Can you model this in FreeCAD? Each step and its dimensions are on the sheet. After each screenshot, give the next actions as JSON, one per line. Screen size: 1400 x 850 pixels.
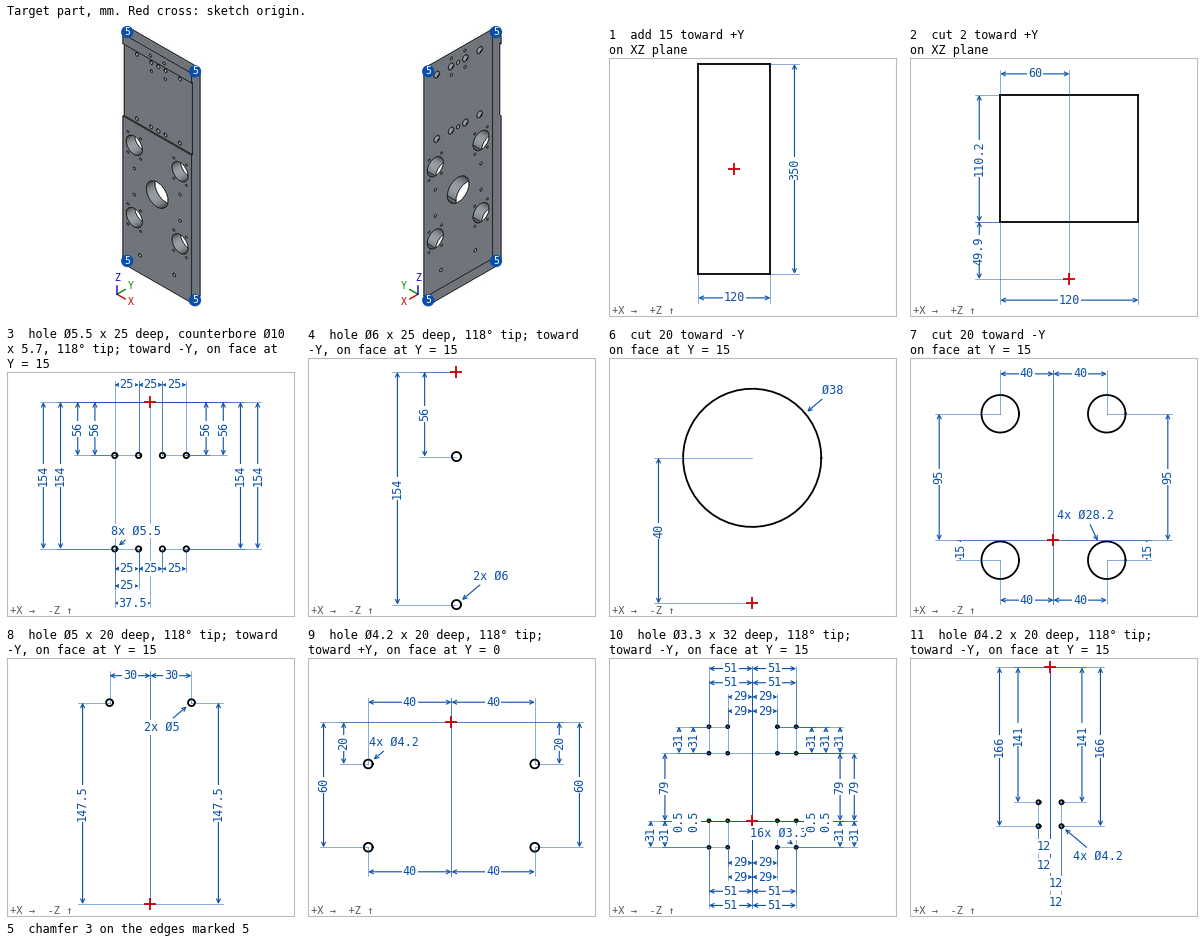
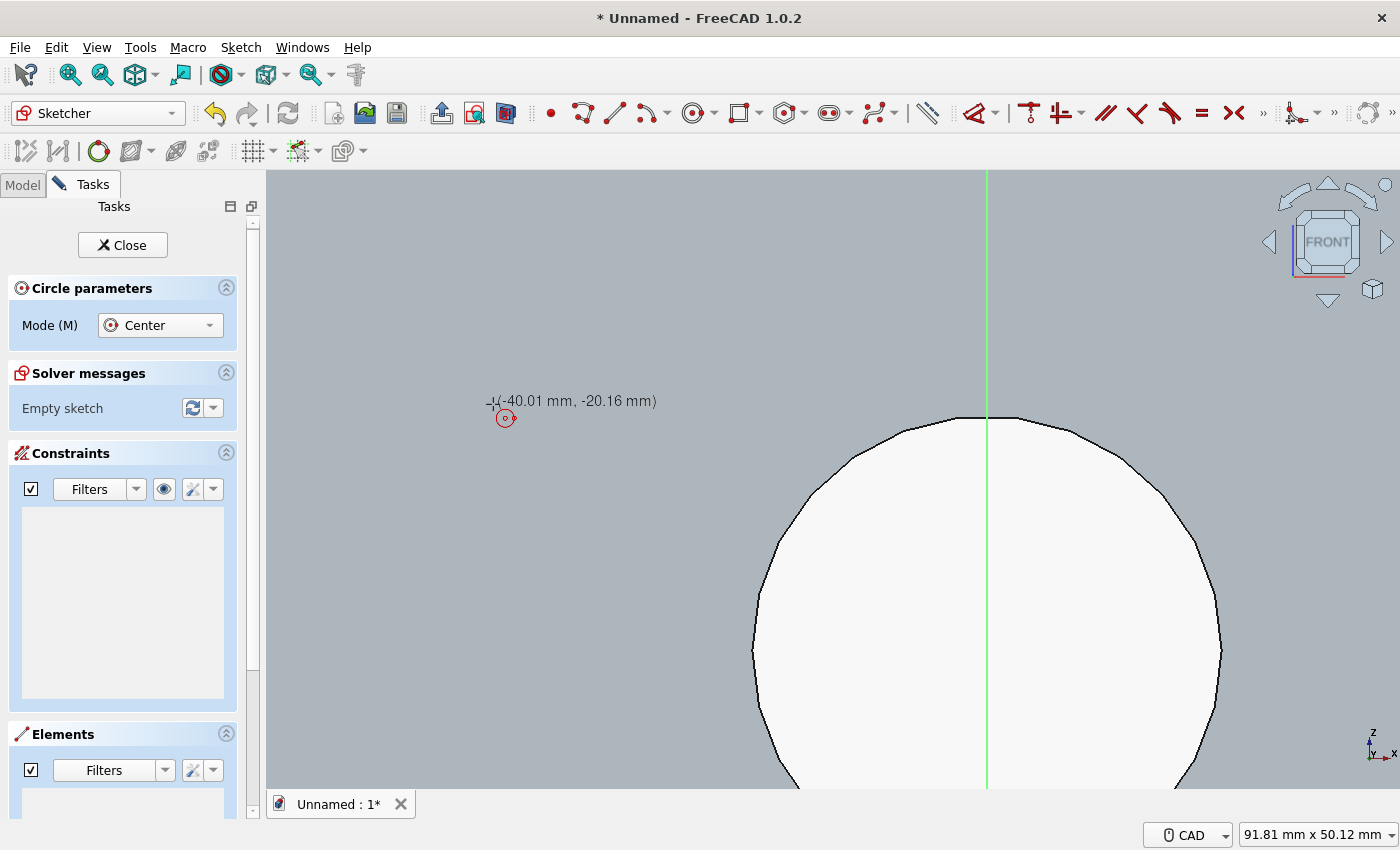
{"action": "left_click", "coordinate": [493, 404]}
{"action": "left_click", "coordinate": [511, 385]}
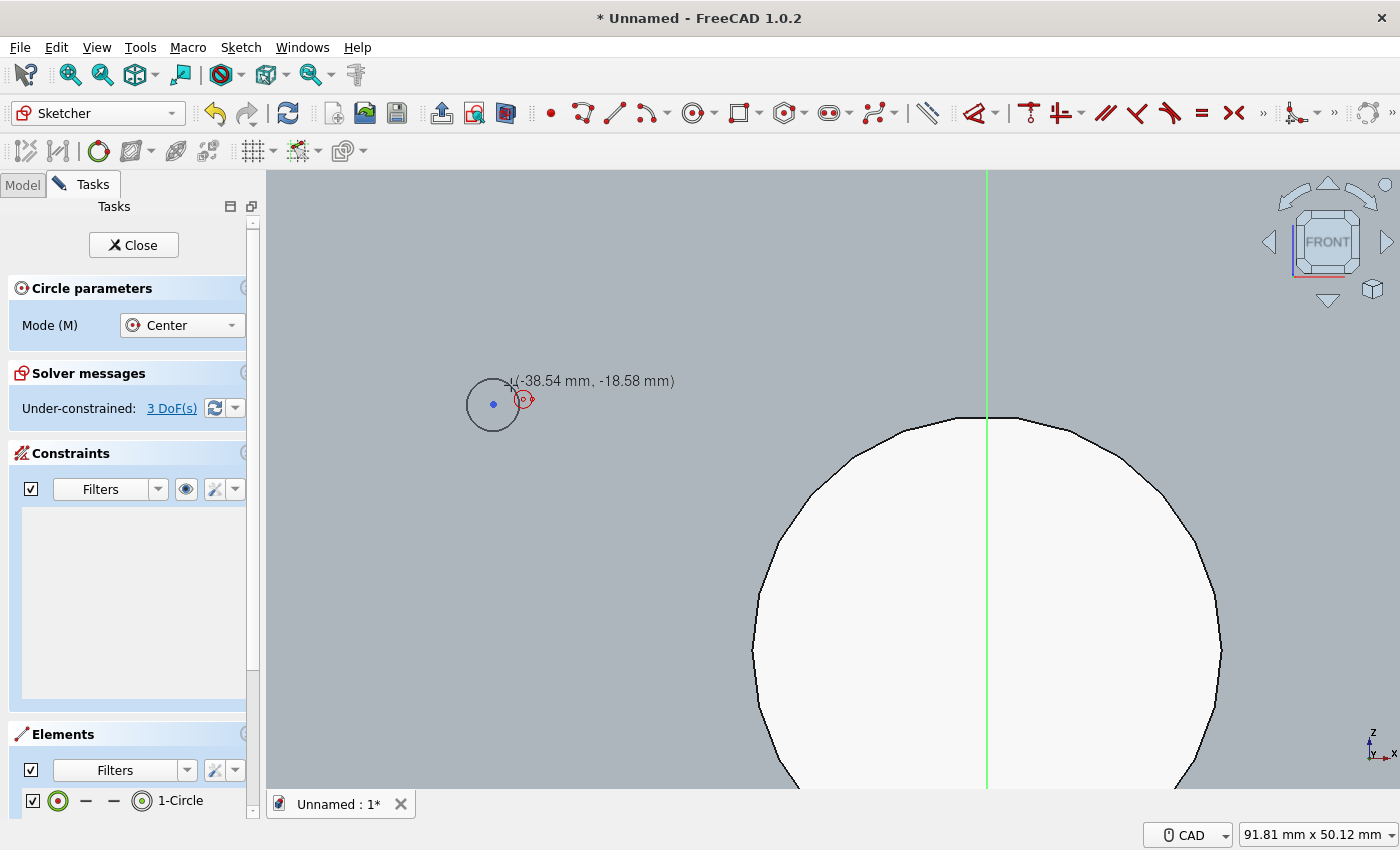
{"action": "scroll", "coordinate": [494, 406], "scroll_direction": "down", "scroll_amount": 3}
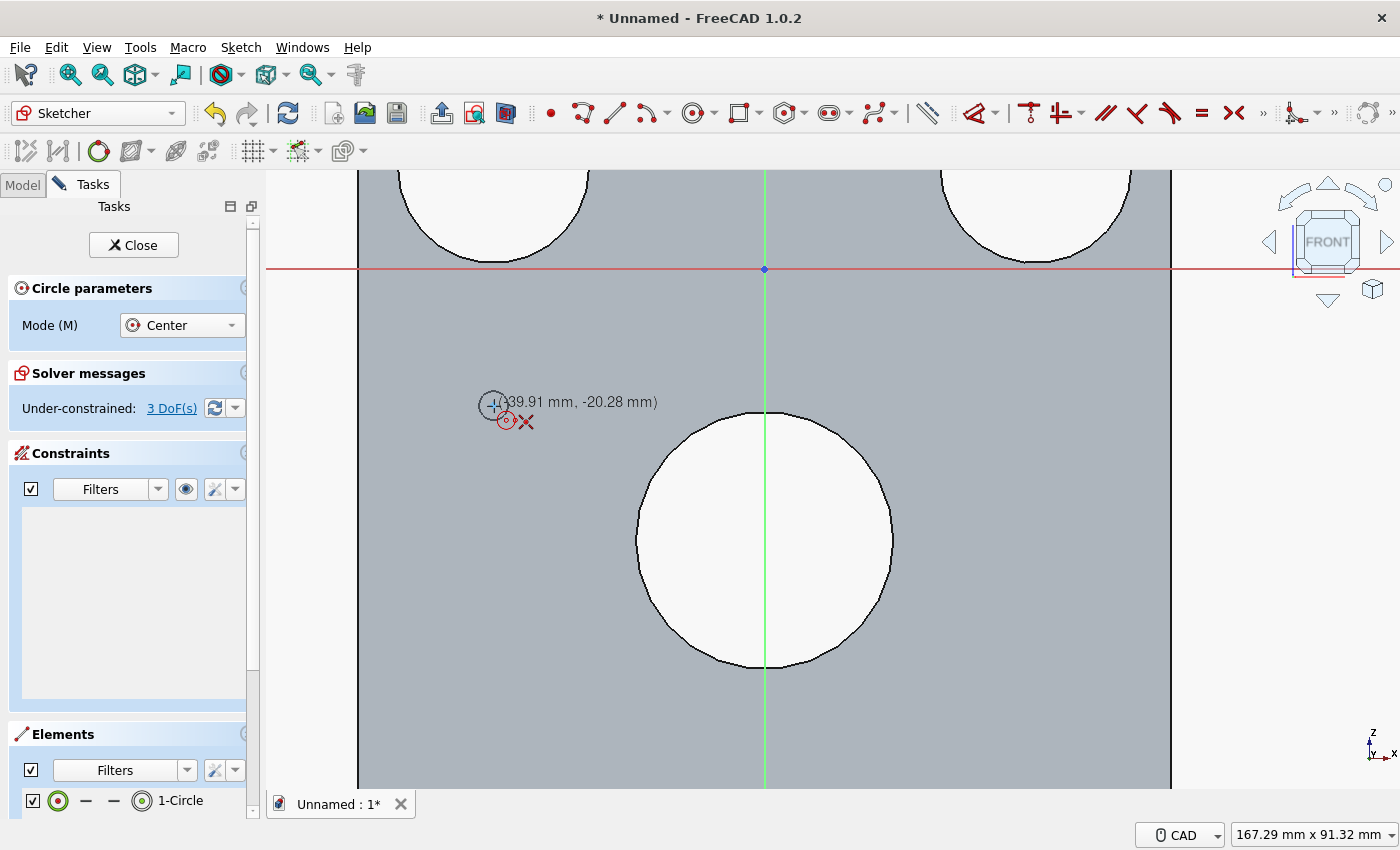
{"action": "scroll", "coordinate": [1036, 405], "scroll_direction": "up", "scroll_amount": 3}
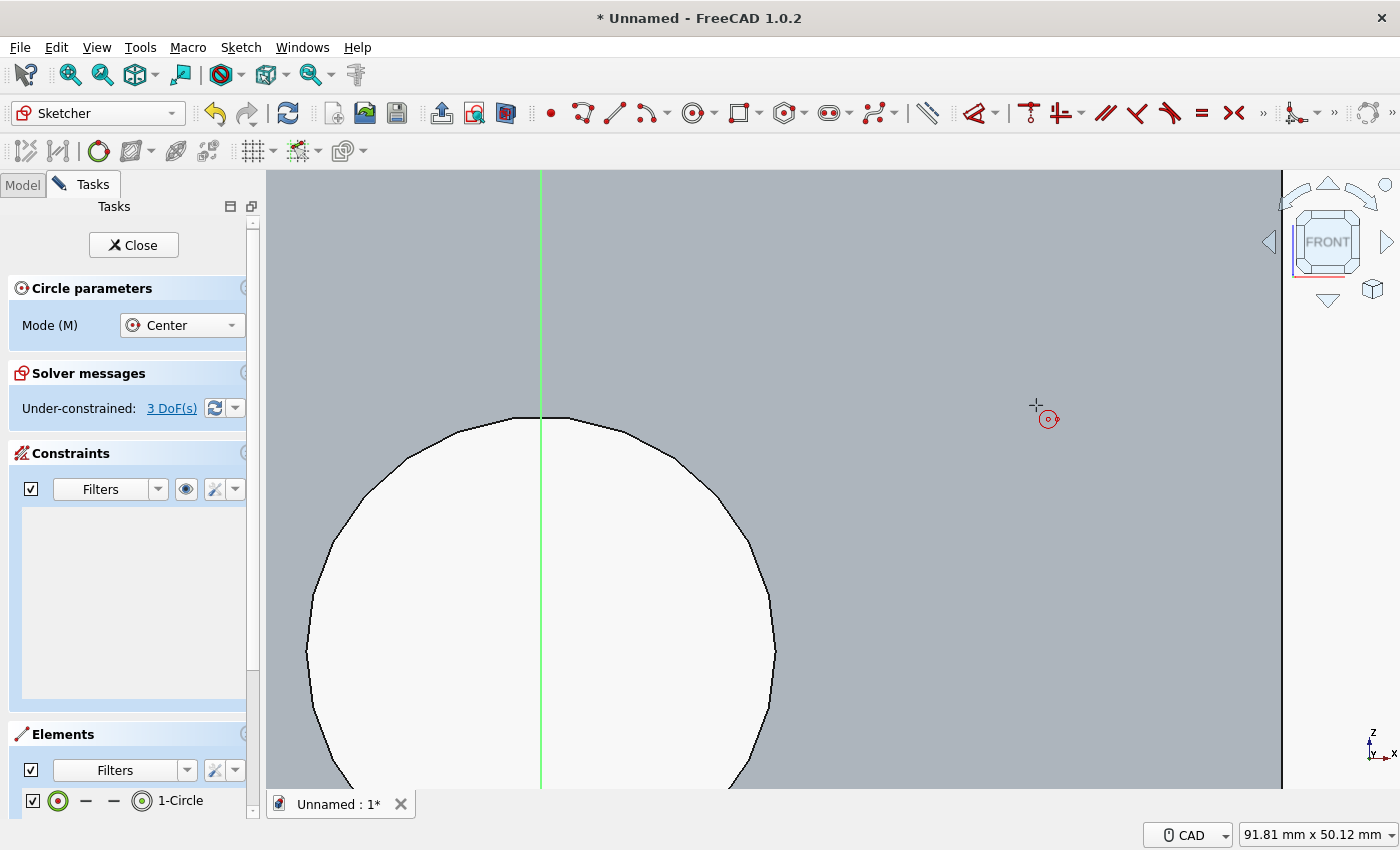
{"action": "left_click", "coordinate": [1035, 404]}
{"action": "left_click", "coordinate": [1053, 386]}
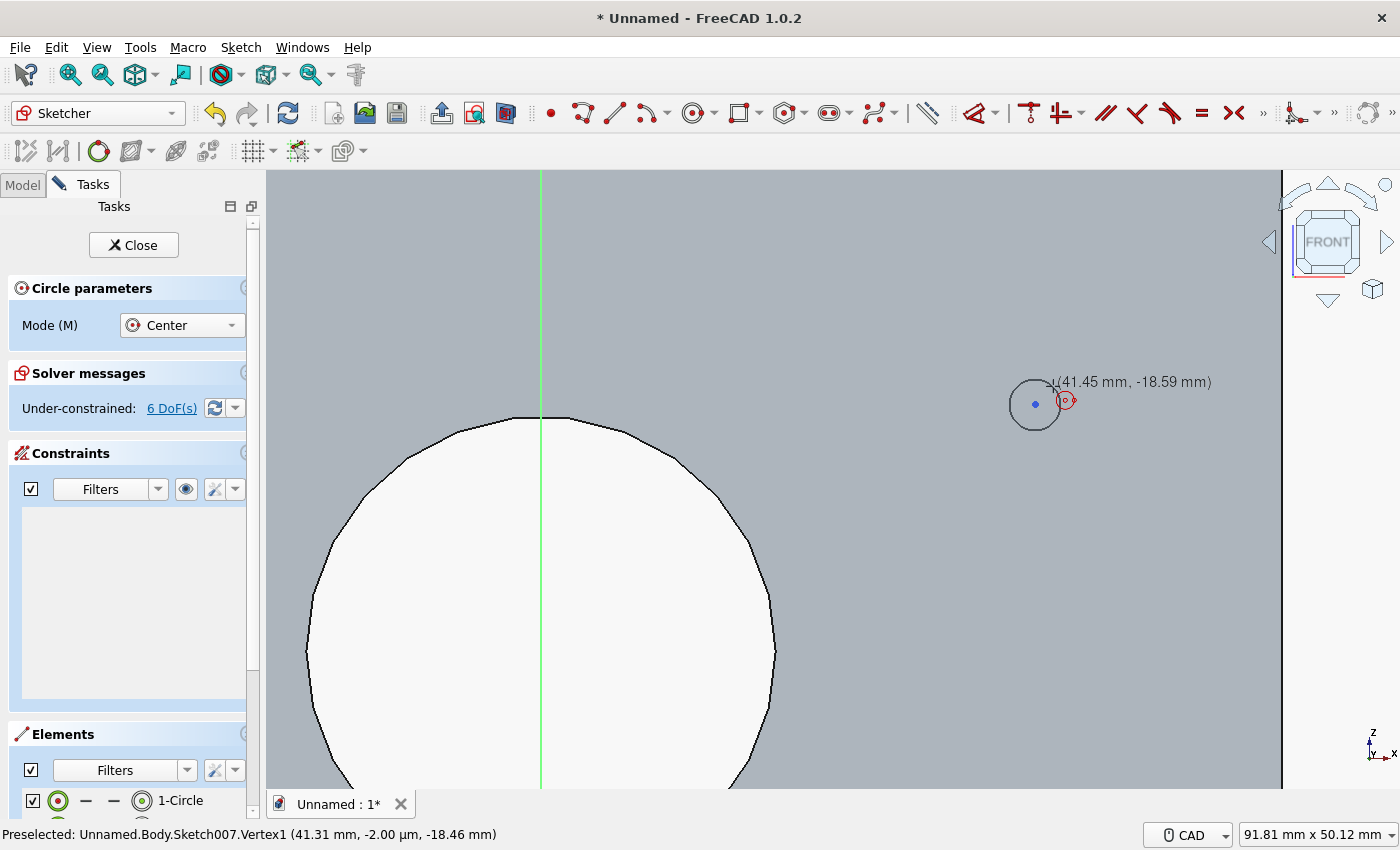
{"action": "scroll", "coordinate": [1036, 405], "scroll_direction": "down", "scroll_amount": 3}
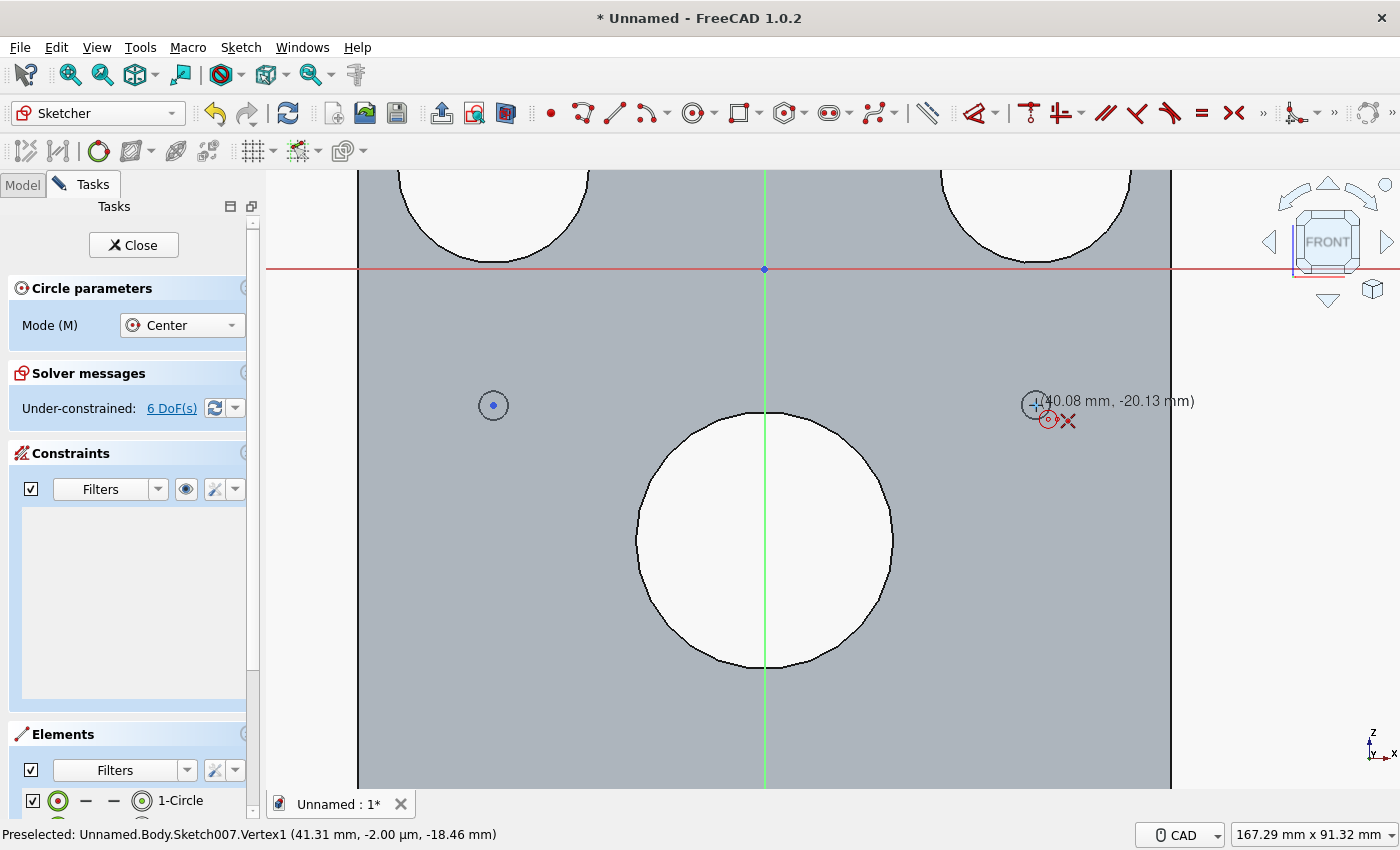
{"action": "scroll", "coordinate": [494, 676], "scroll_direction": "up", "scroll_amount": 3}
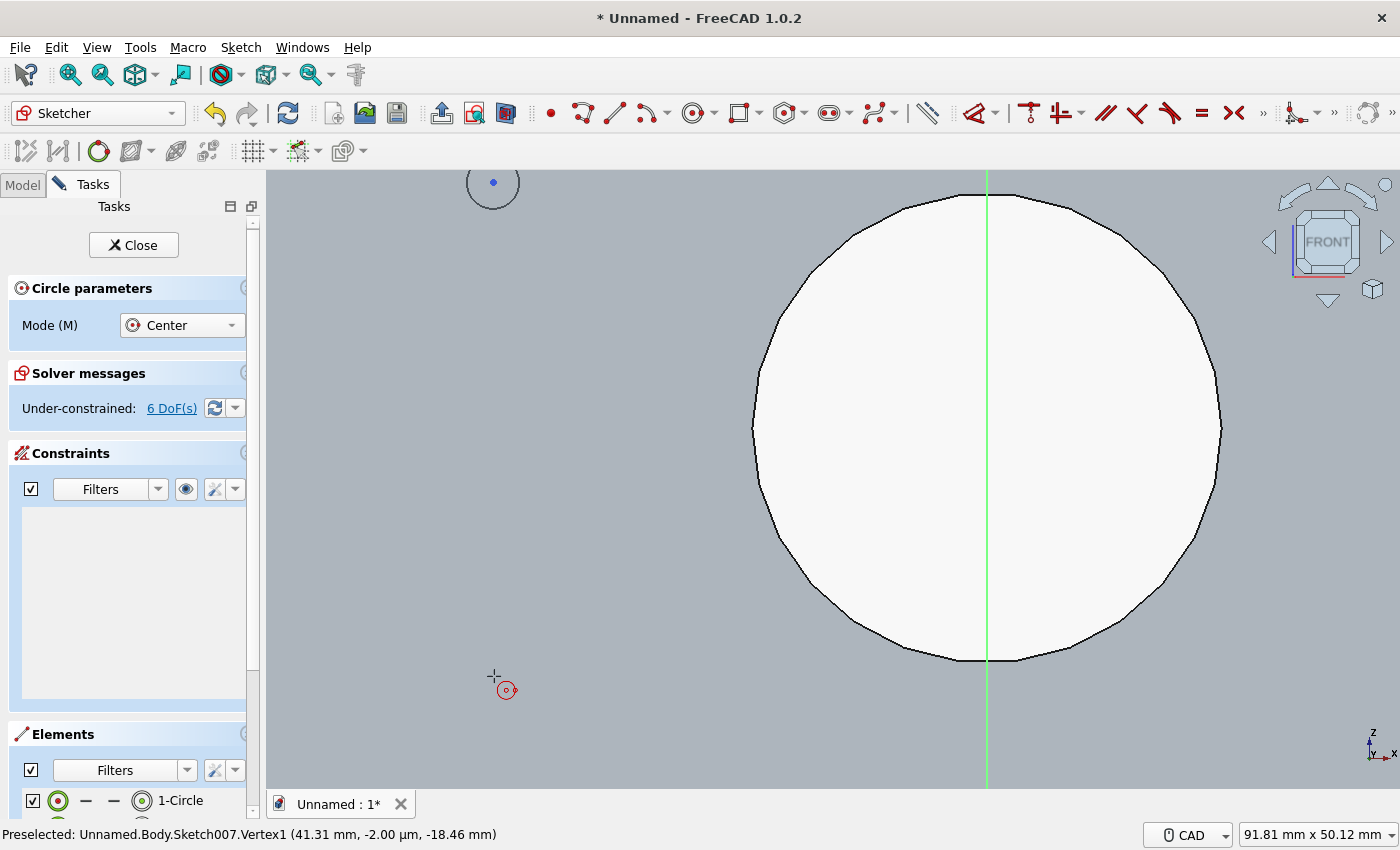
{"action": "left_click", "coordinate": [493, 675]}
{"action": "left_click", "coordinate": [511, 657]}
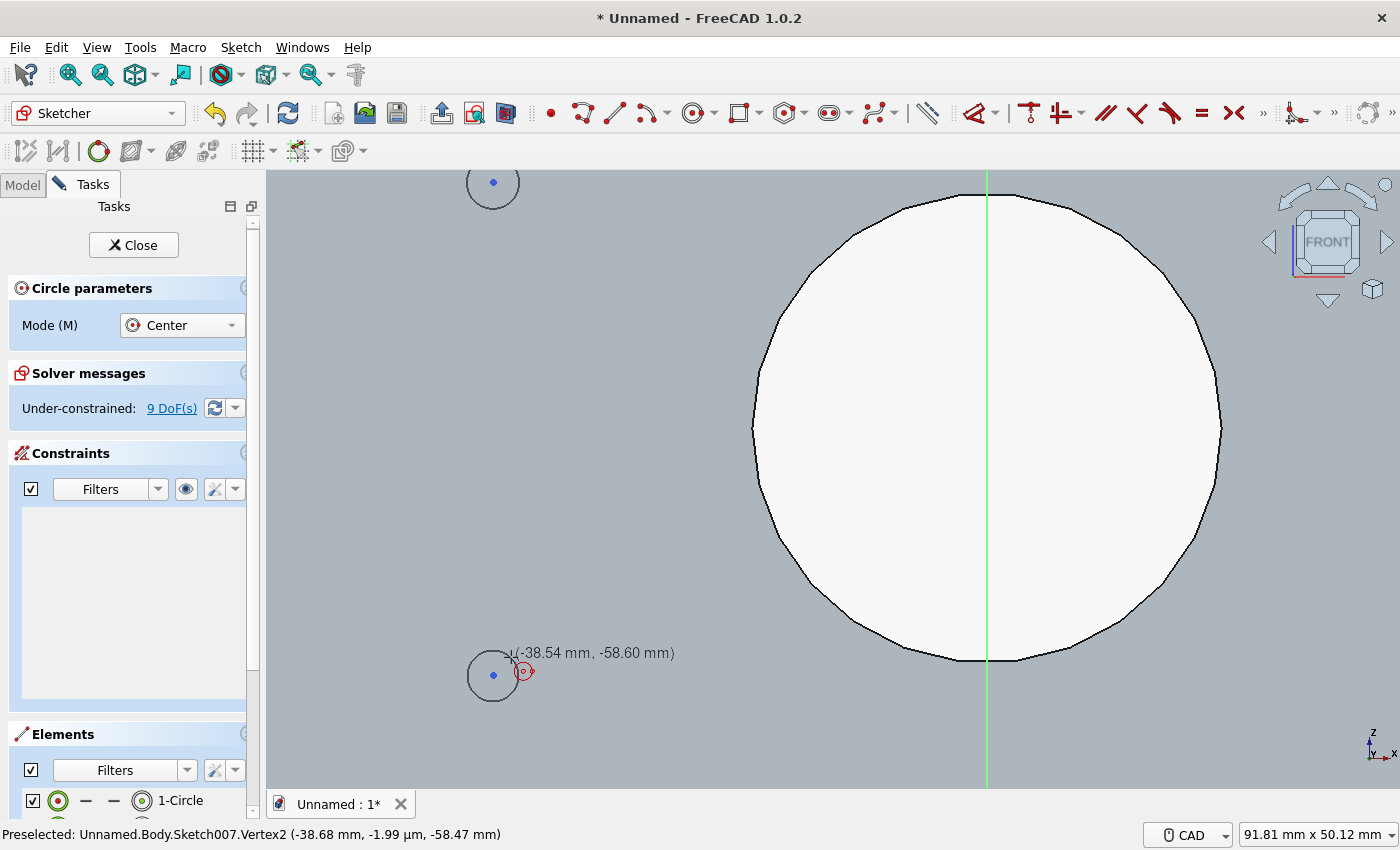
{"action": "scroll", "coordinate": [494, 676], "scroll_direction": "down", "scroll_amount": 3}